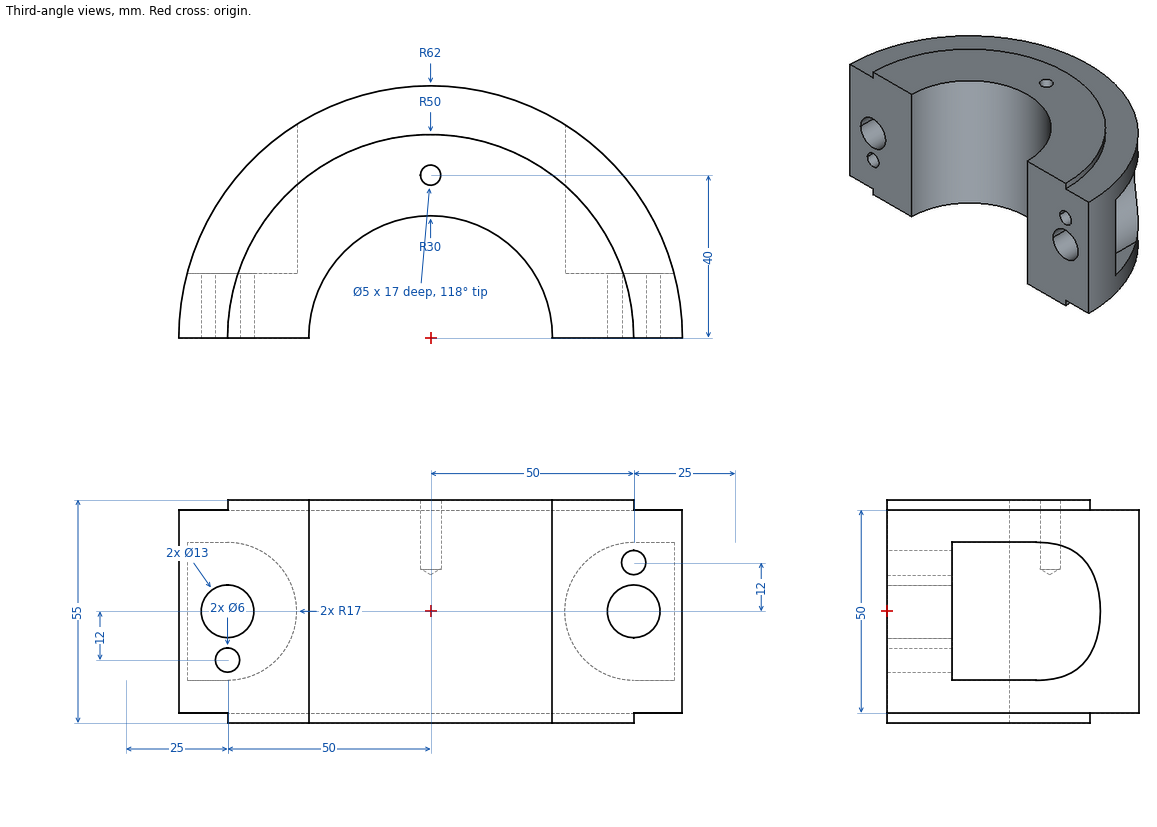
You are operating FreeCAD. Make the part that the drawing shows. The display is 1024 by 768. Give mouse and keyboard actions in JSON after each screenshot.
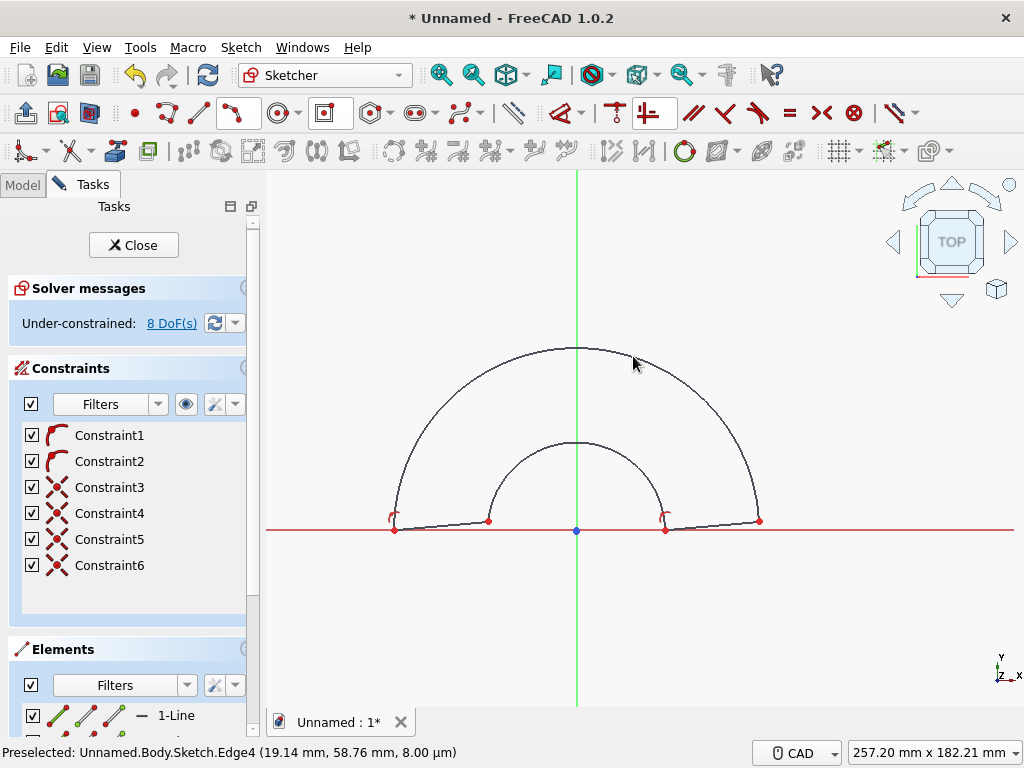
{"action": "left_click", "coordinate": [422, 528]}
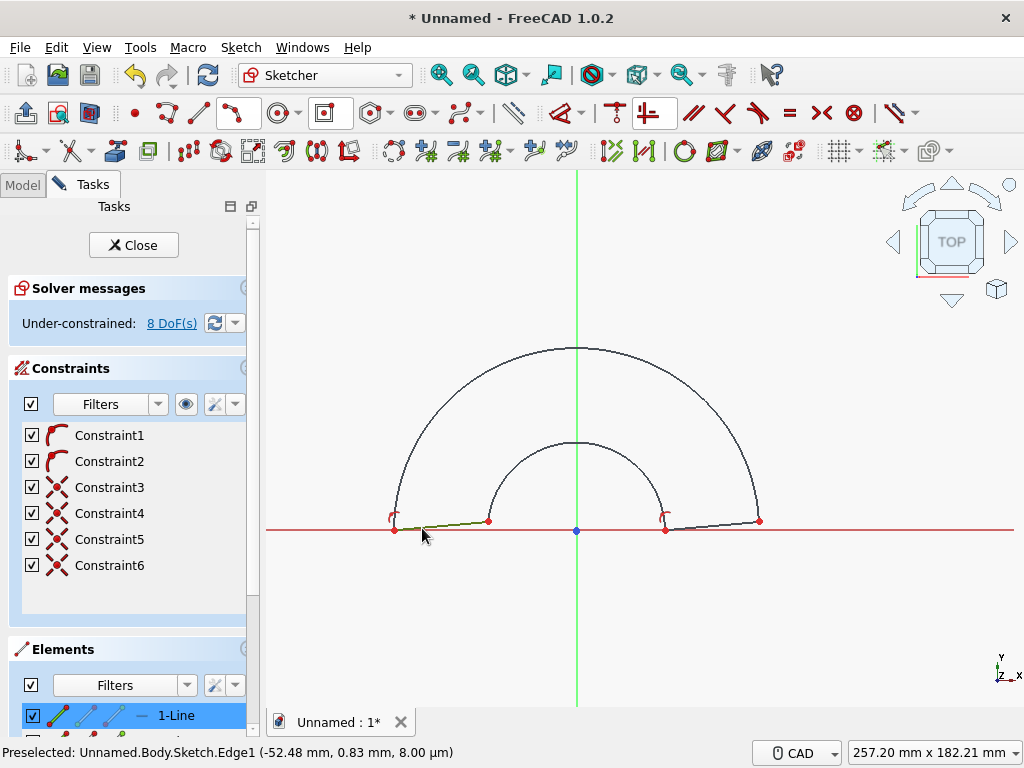
{"action": "key", "text": "h"}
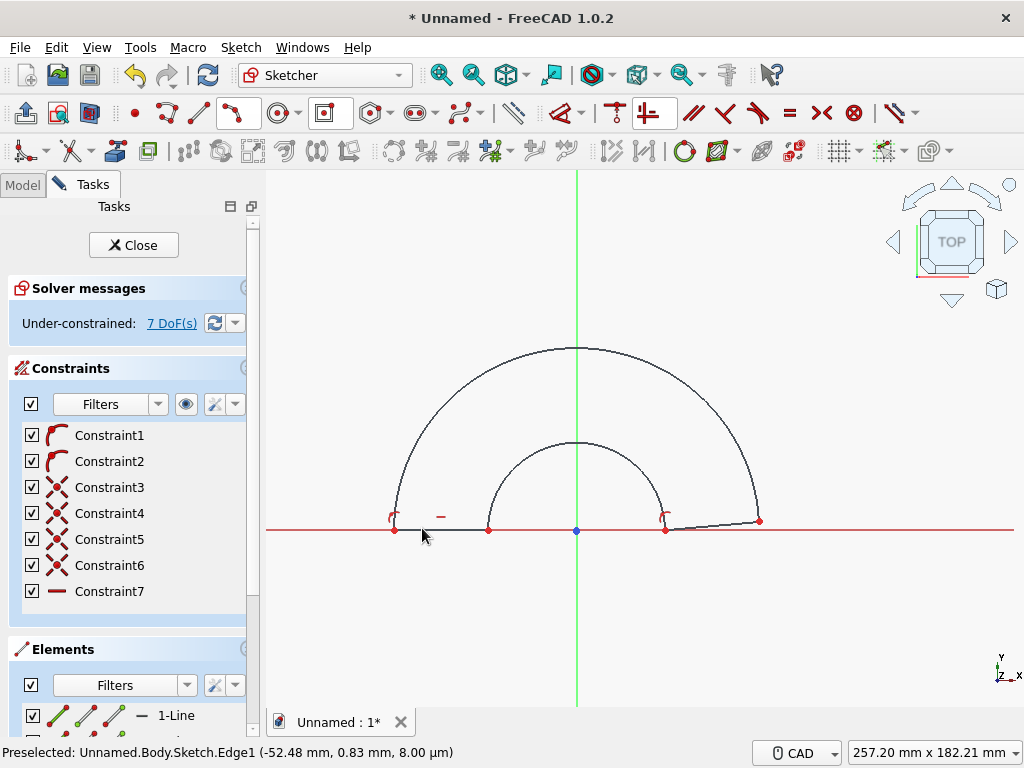
{"action": "left_click", "coordinate": [693, 528]}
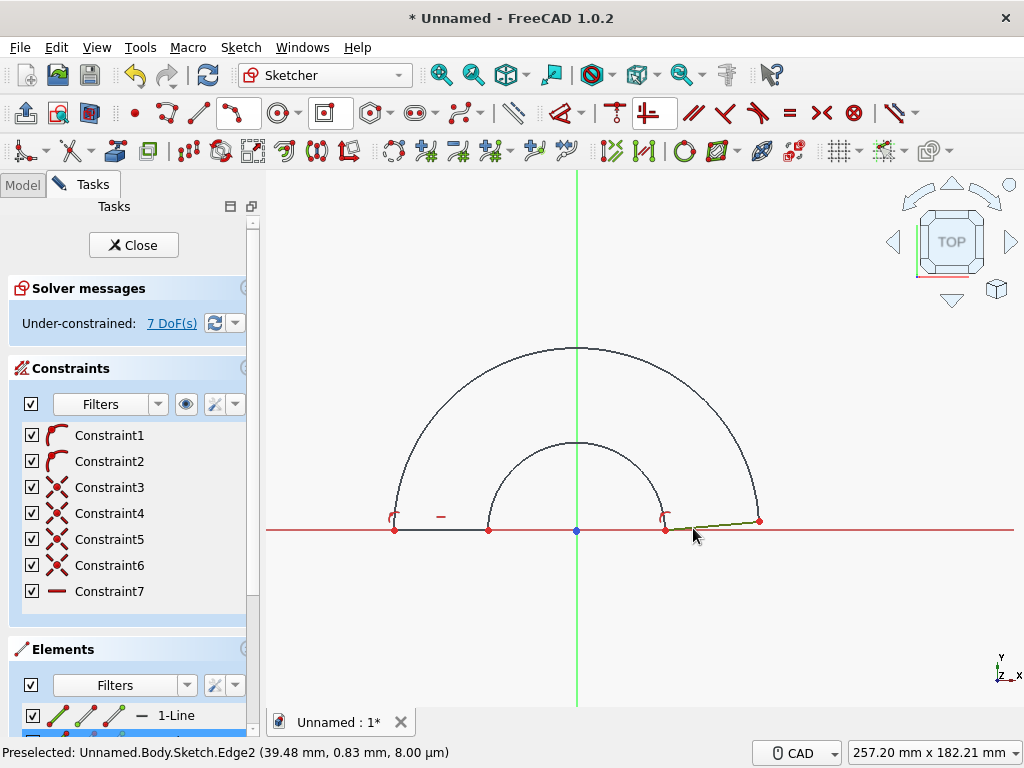
{"action": "key", "text": "h"}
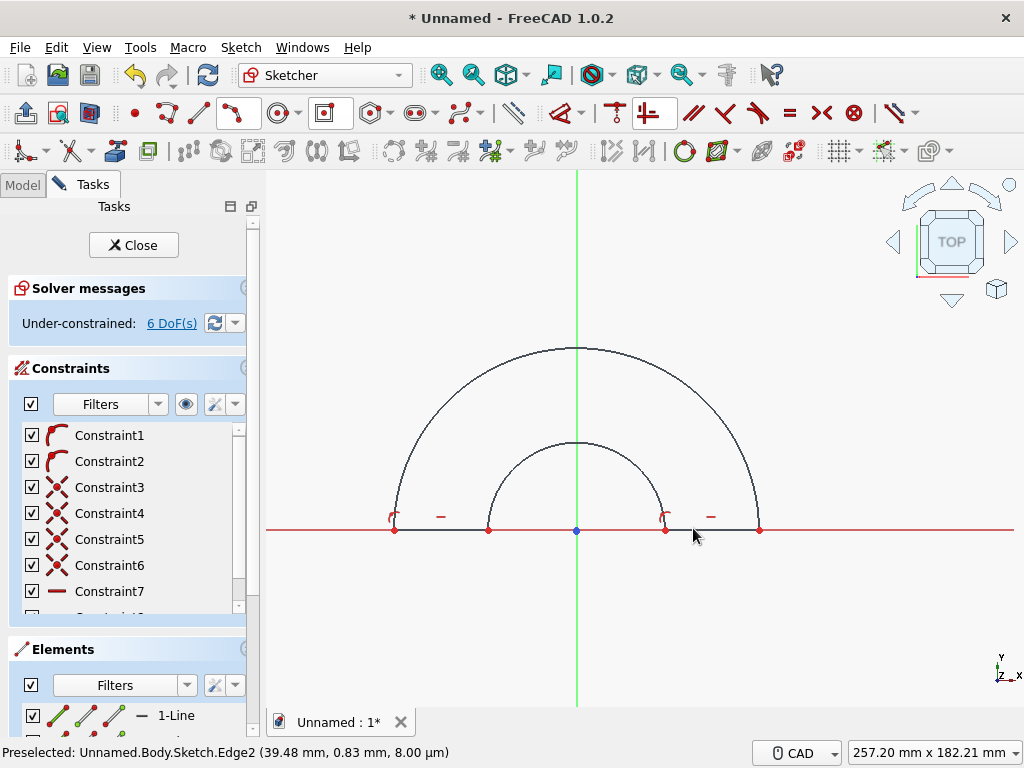
{"action": "left_click", "coordinate": [628, 459]}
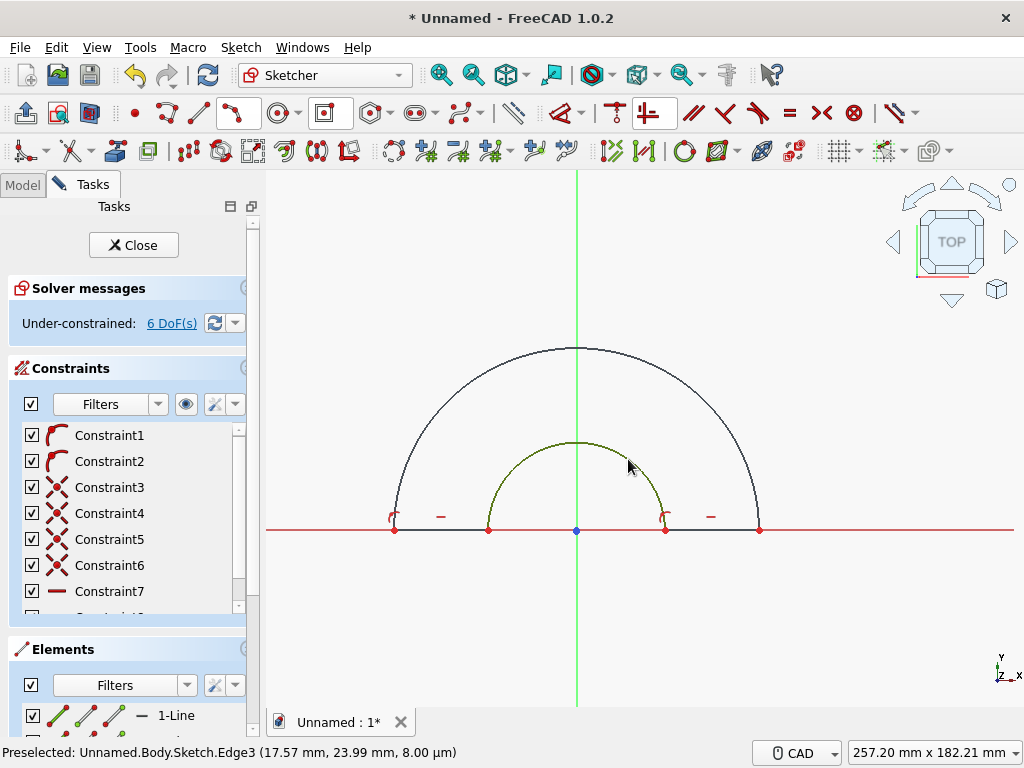
{"action": "left_click", "coordinate": [684, 383]}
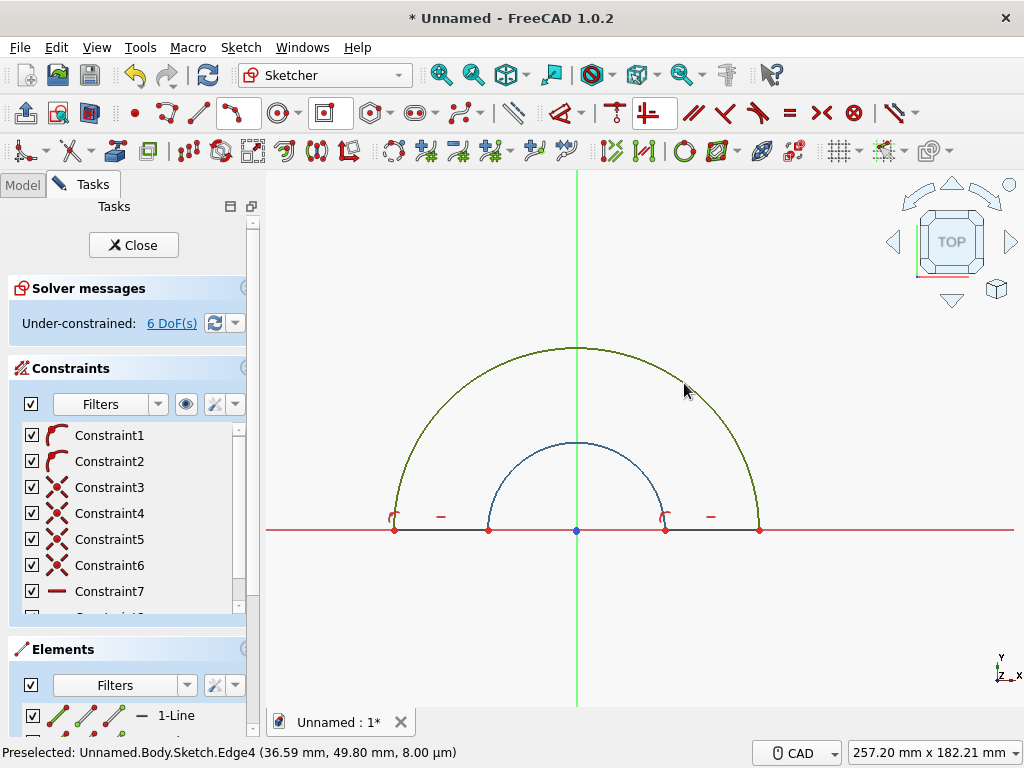
{"action": "left_click", "coordinate": [616, 114]}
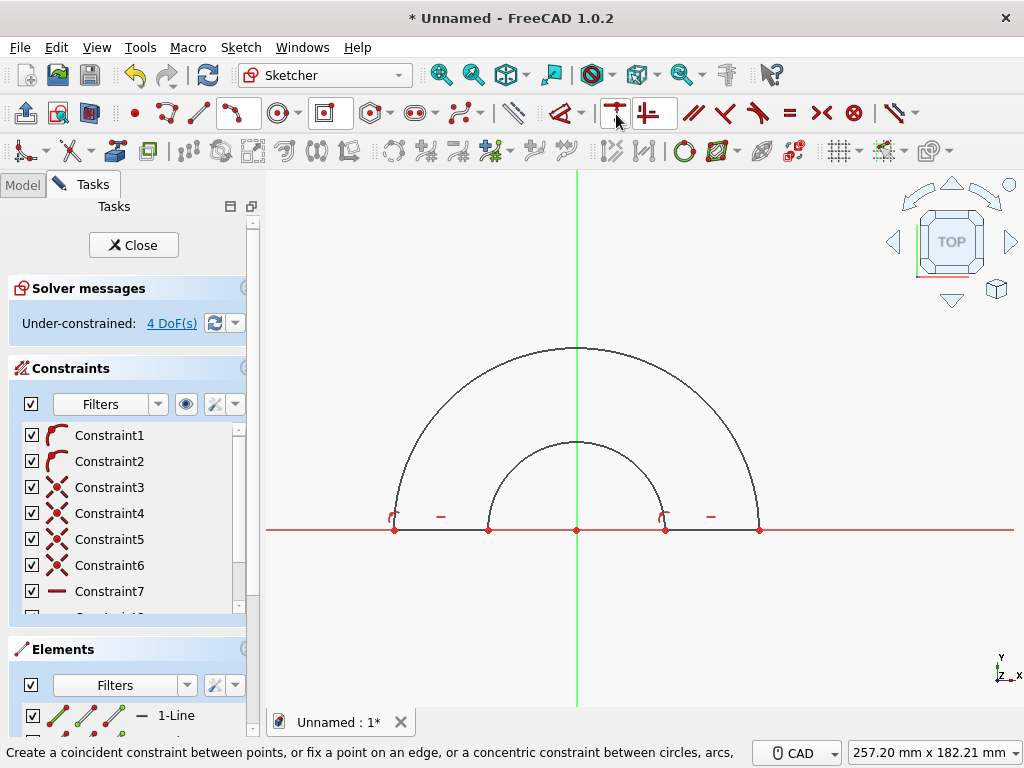
{"action": "left_click_drag", "start_coordinate": [566, 520], "coordinate": [587, 541]}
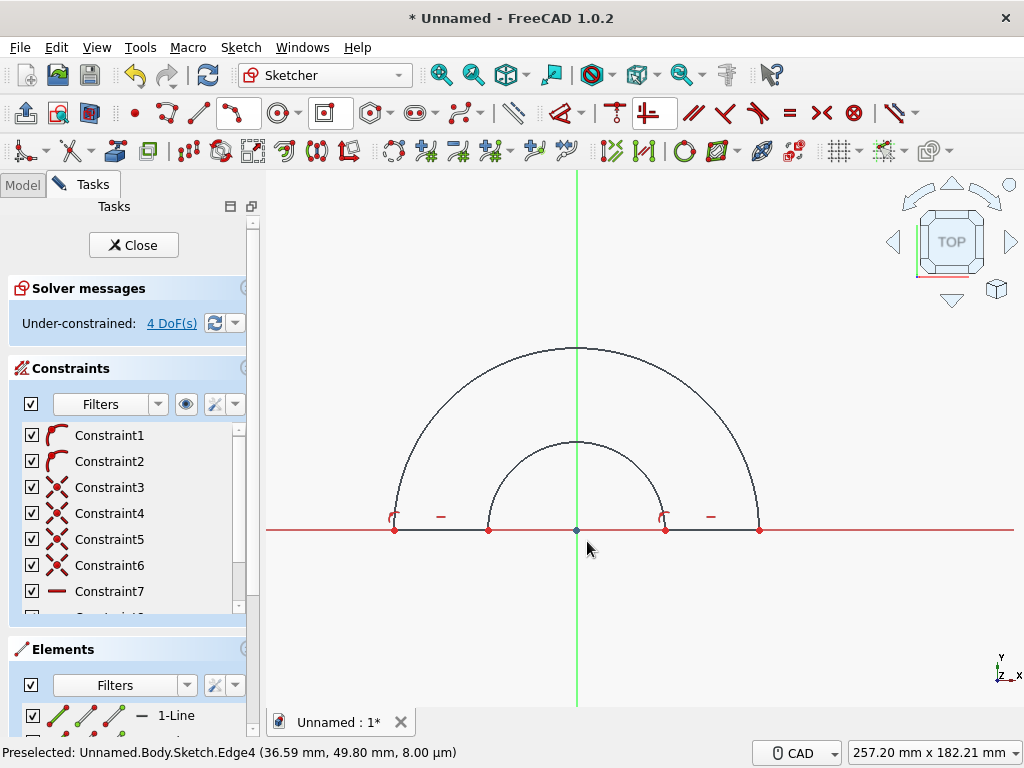
{"action": "left_click", "coordinate": [616, 114]}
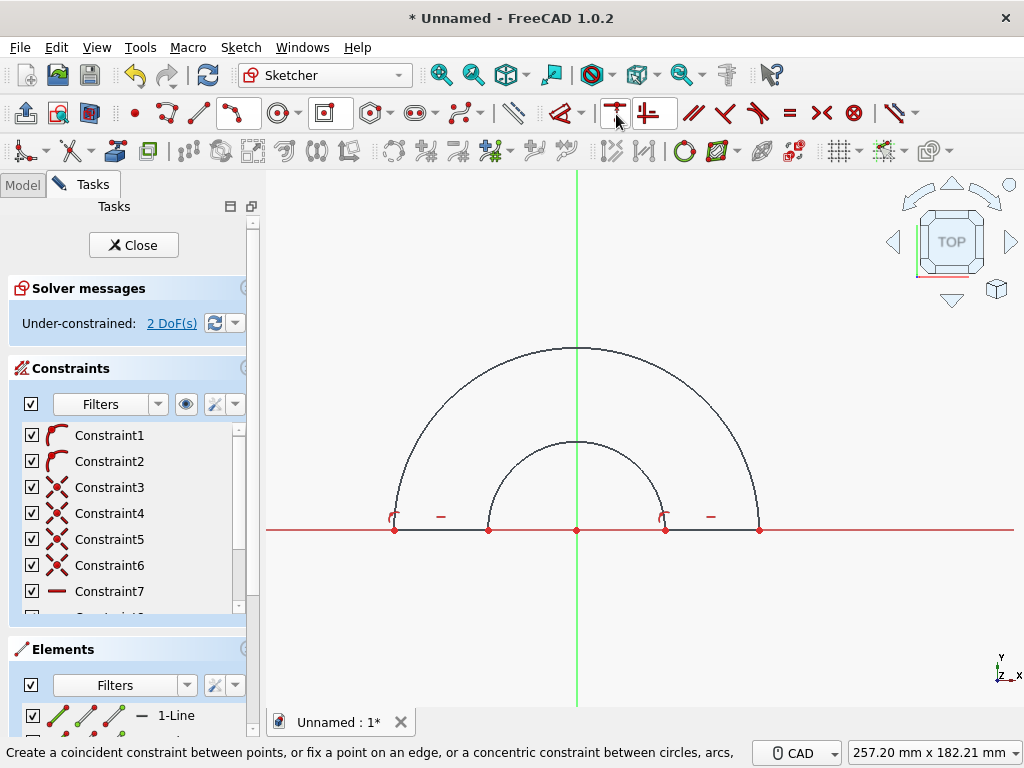
{"action": "left_click", "coordinate": [560, 114]}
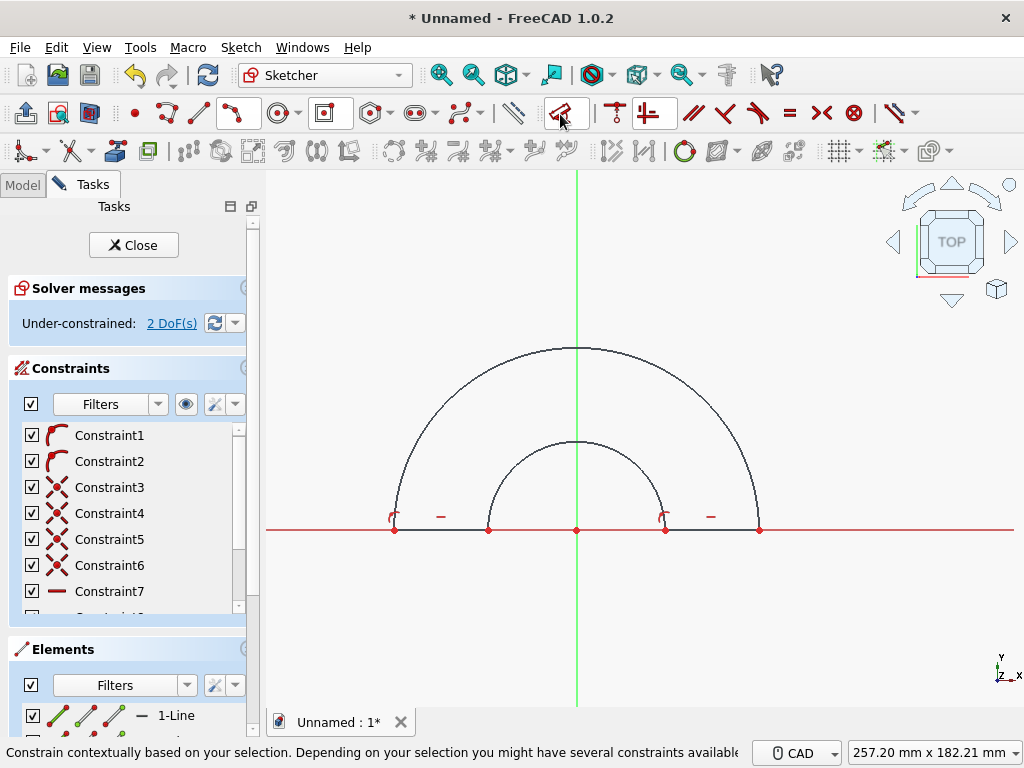
{"action": "left_click", "coordinate": [629, 459]}
{"action": "left_click", "coordinate": [648, 433]}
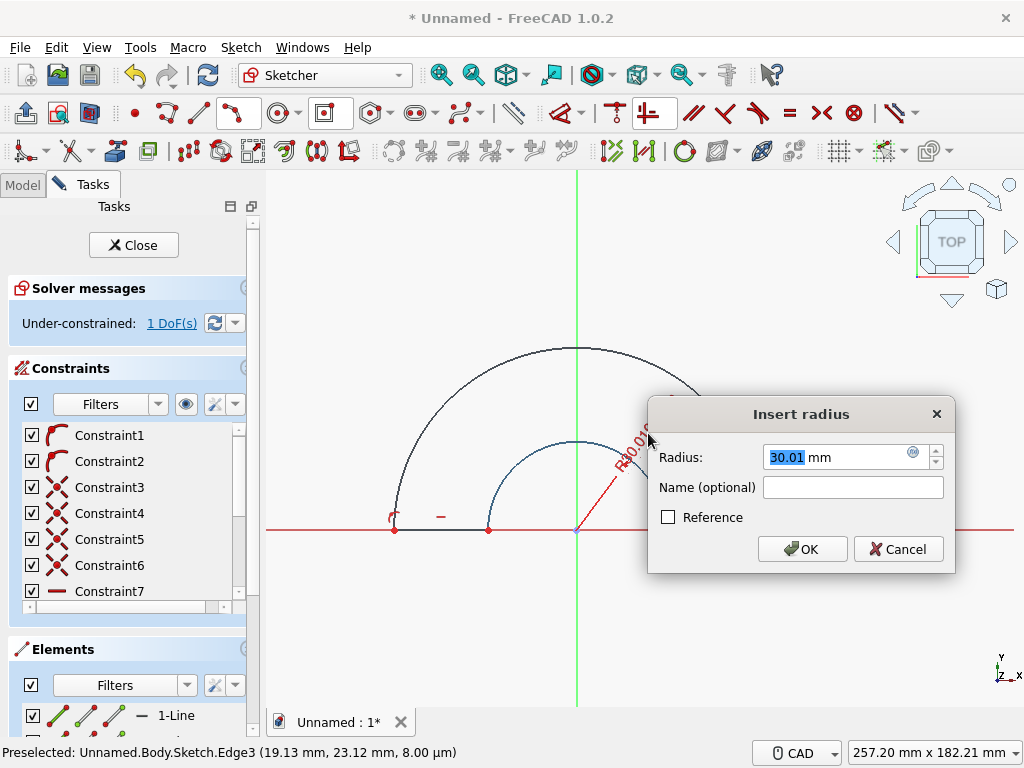
{"action": "type", "text": "30"}
{"action": "key", "text": "Return"}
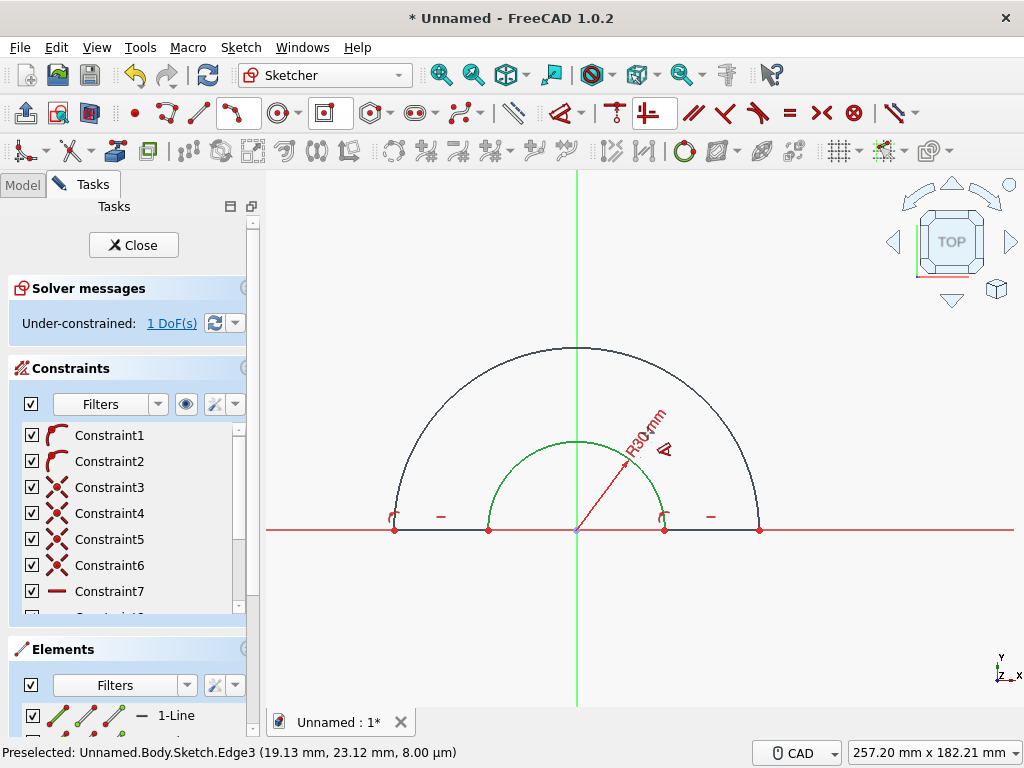
{"action": "left_click", "coordinate": [684, 383]}
{"action": "left_click", "coordinate": [703, 357]}